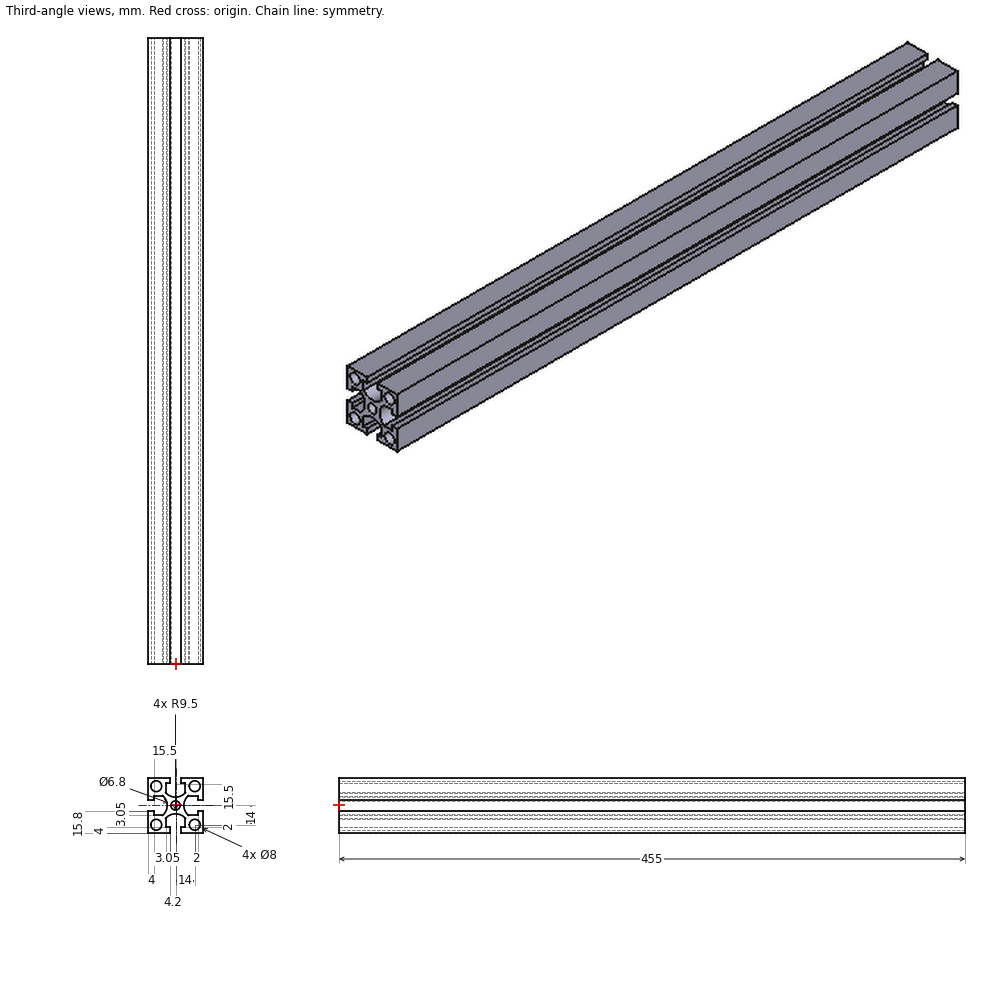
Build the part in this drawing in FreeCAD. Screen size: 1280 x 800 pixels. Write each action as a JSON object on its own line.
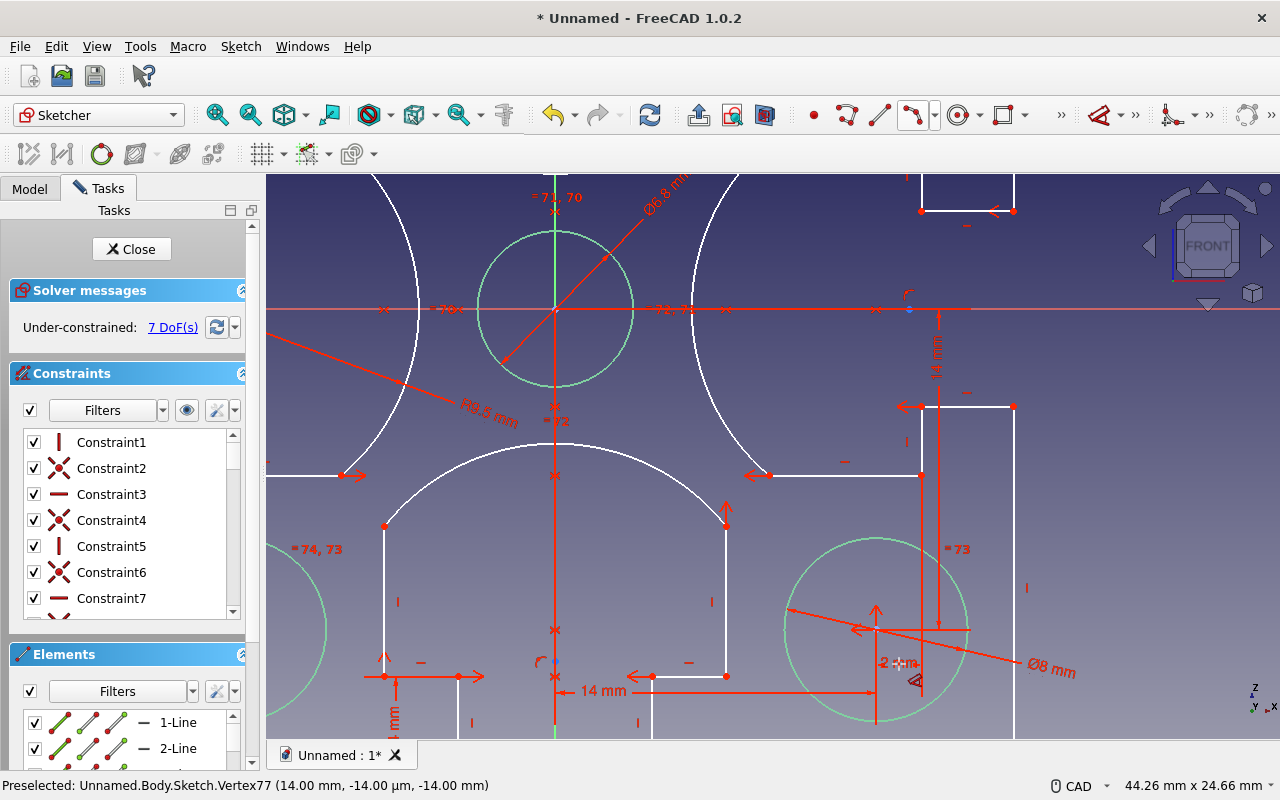
{"action": "left_click", "coordinate": [726, 677]}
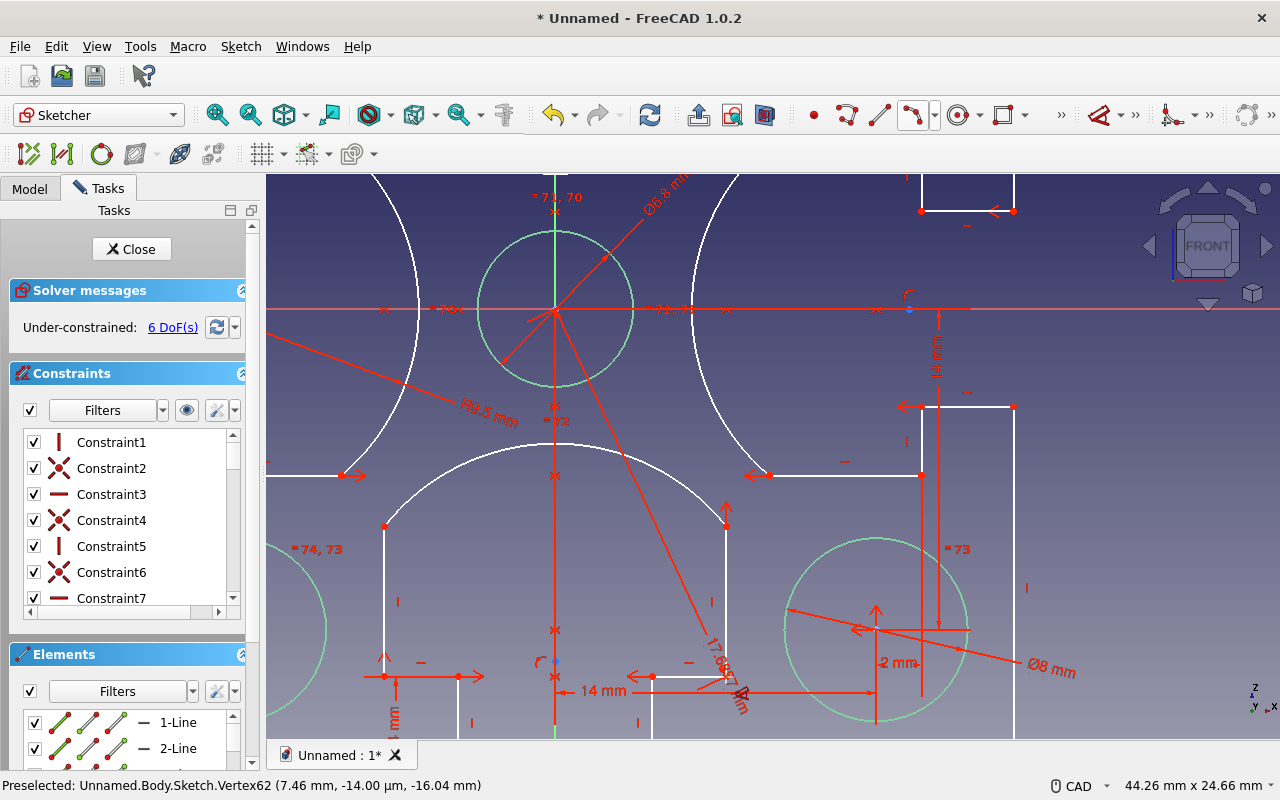
{"action": "left_click", "coordinate": [876, 630]}
{"action": "left_click", "coordinate": [910, 642]}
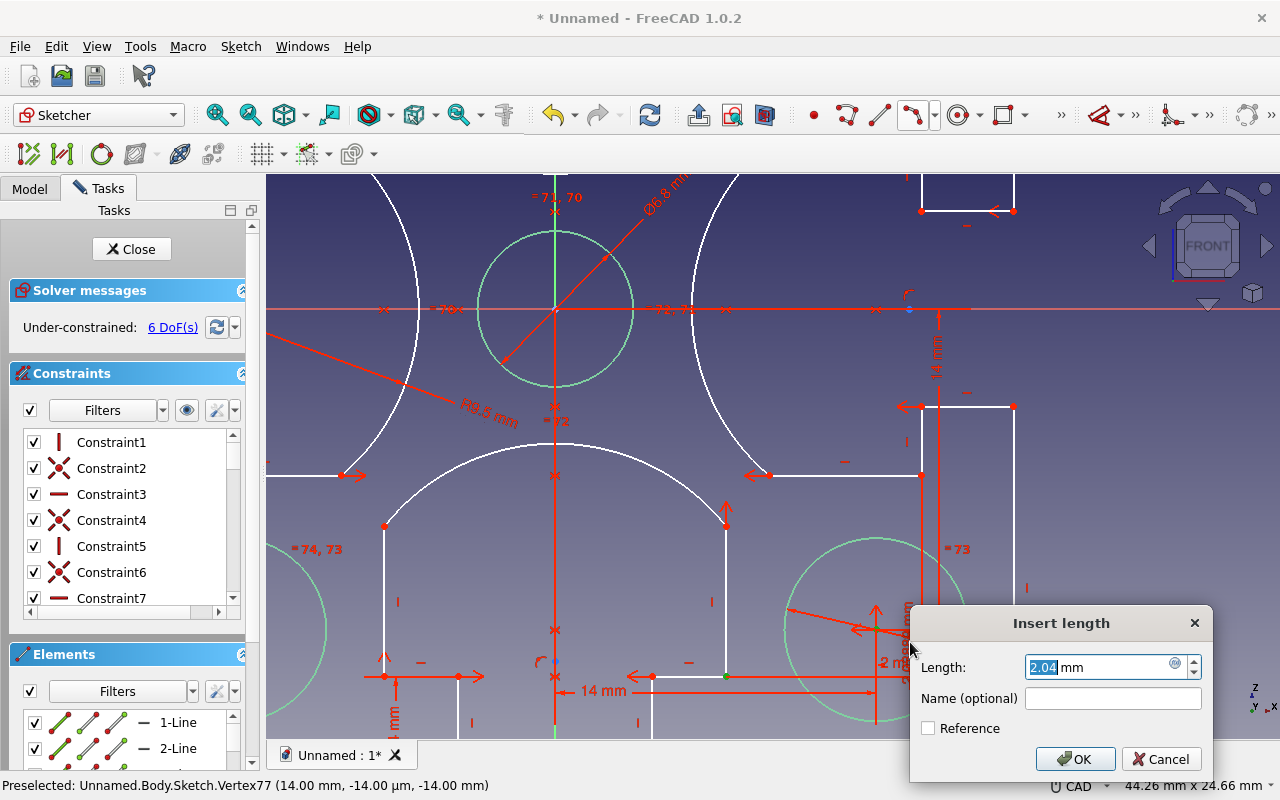
{"action": "type", "text": "2"}
{"action": "key", "text": "Return"}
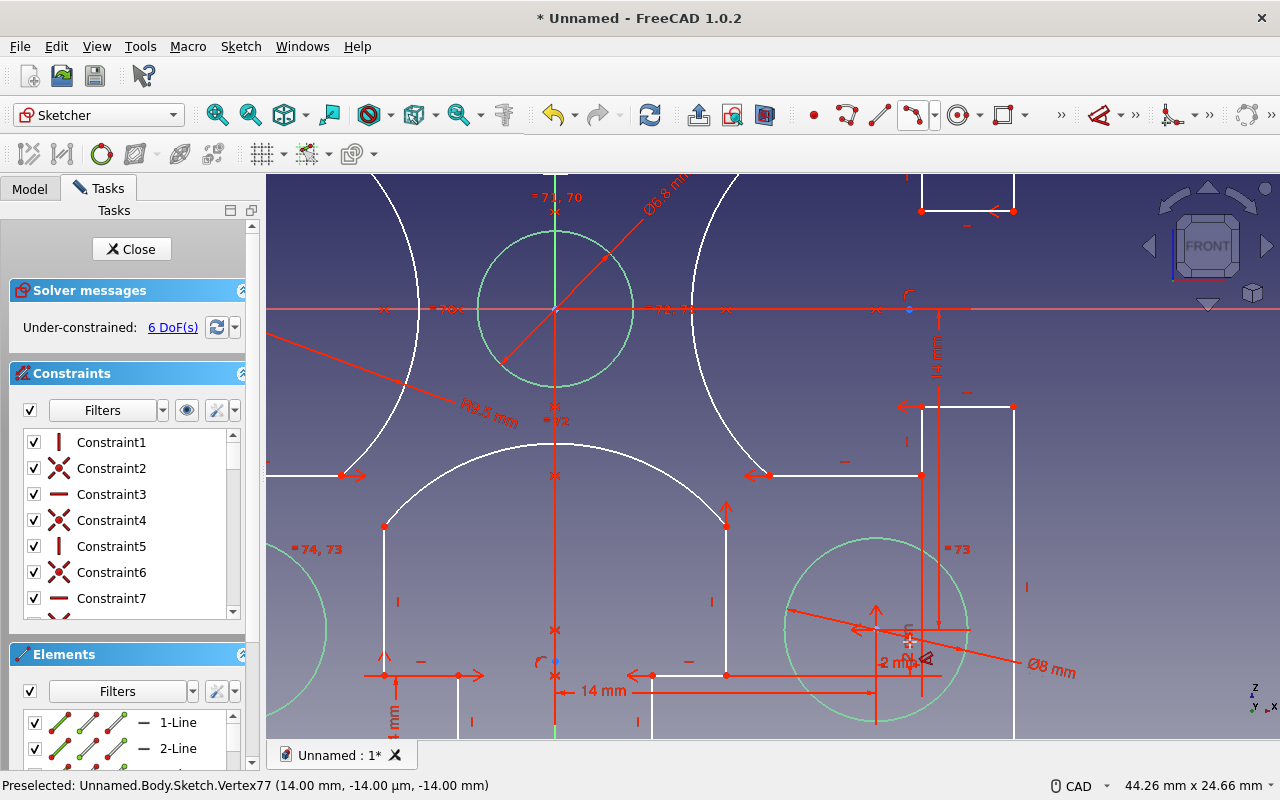
{"action": "left_click", "coordinate": [407, 676]}
{"action": "left_click", "coordinate": [421, 642]}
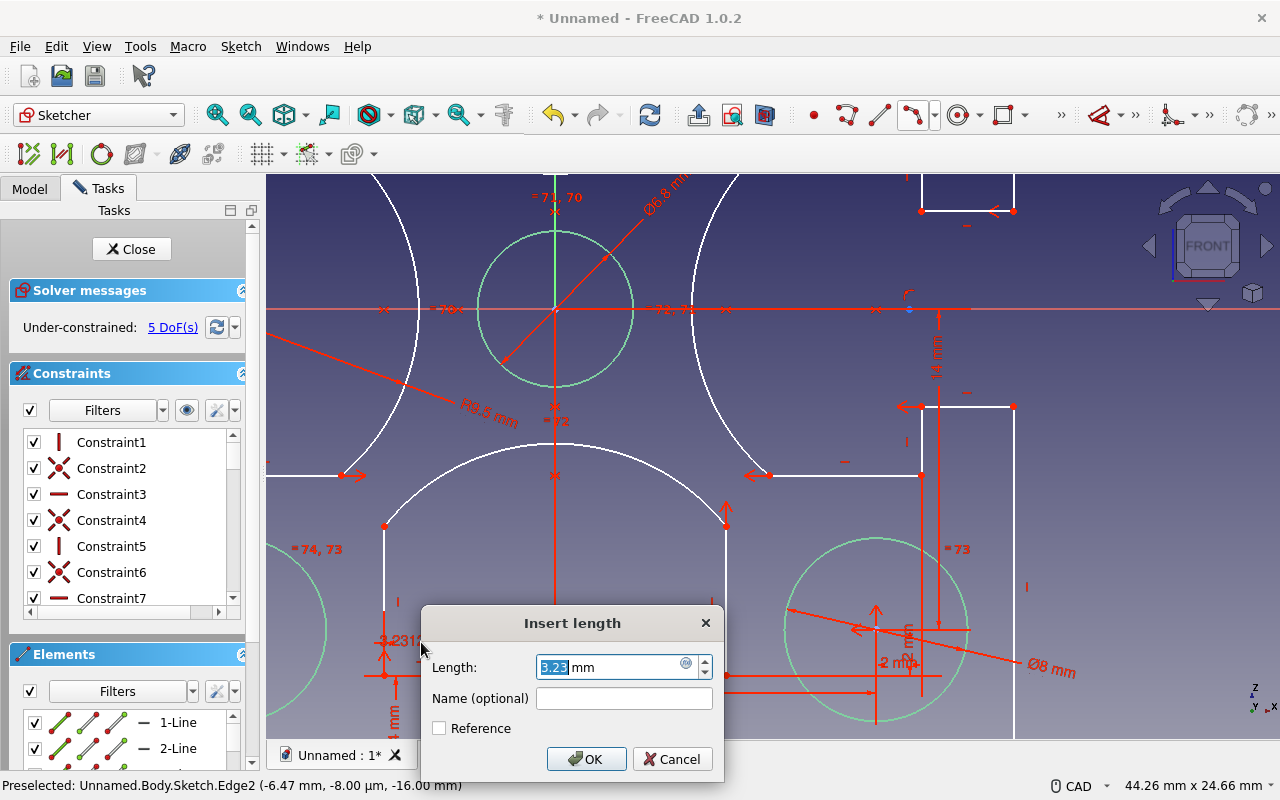
{"action": "type", "text": "3.05"}
{"action": "key", "text": "Return"}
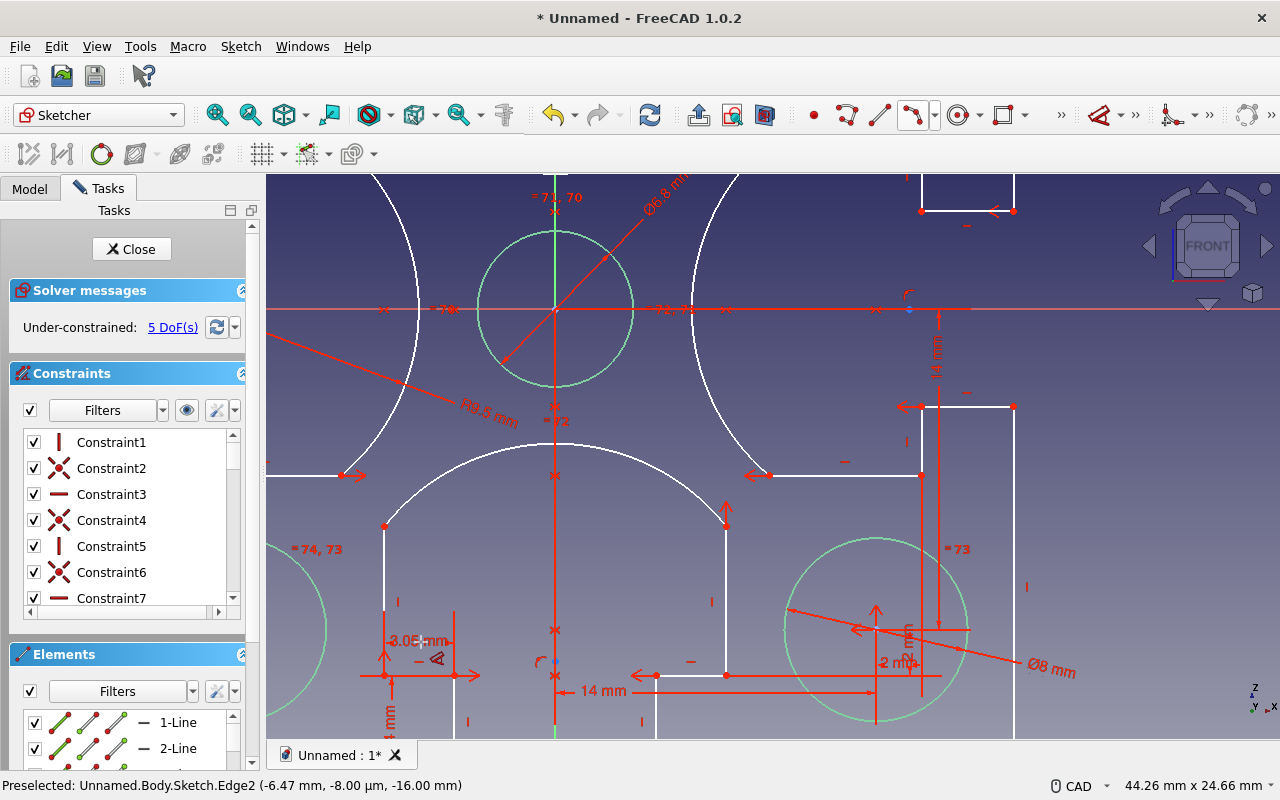
{"action": "scroll", "coordinate": [791, 542], "scroll_direction": "down", "scroll_amount": 5}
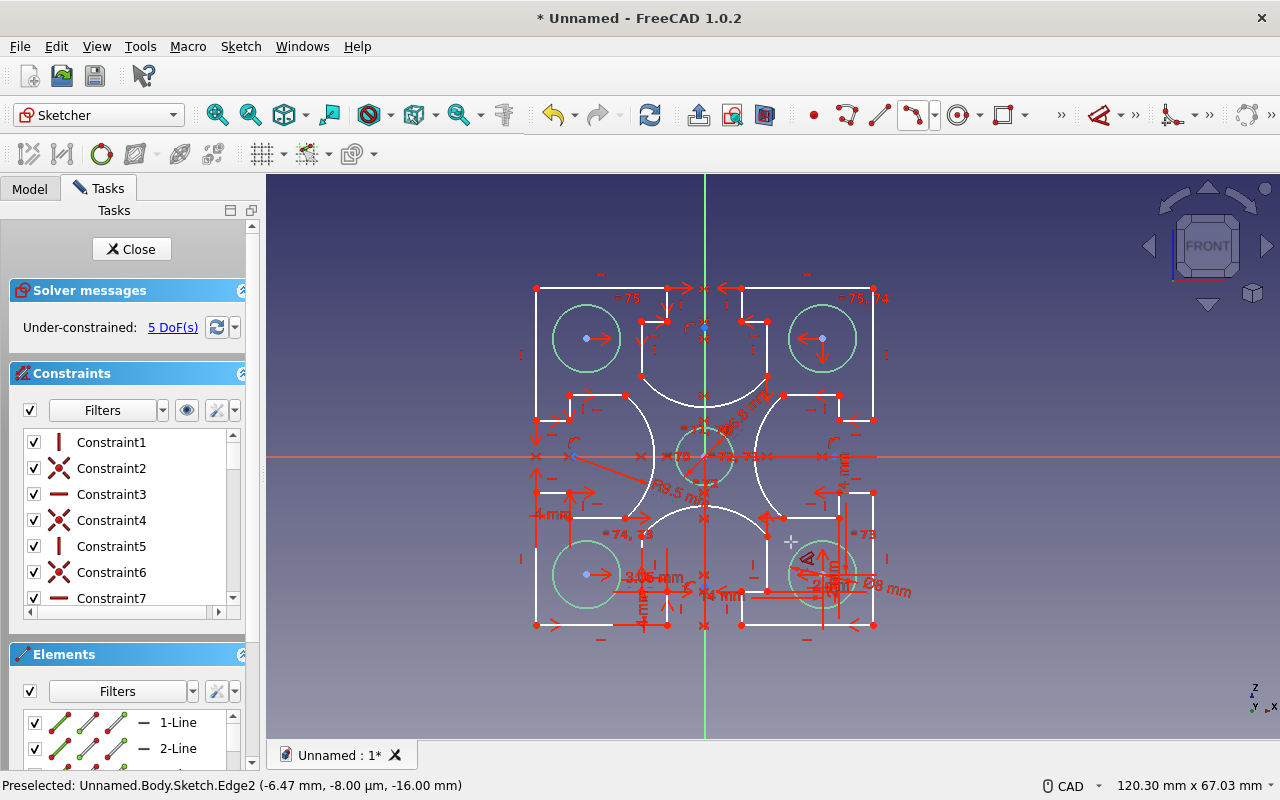
{"action": "left_click", "coordinate": [536, 585]}
{"action": "left_click", "coordinate": [502, 559]}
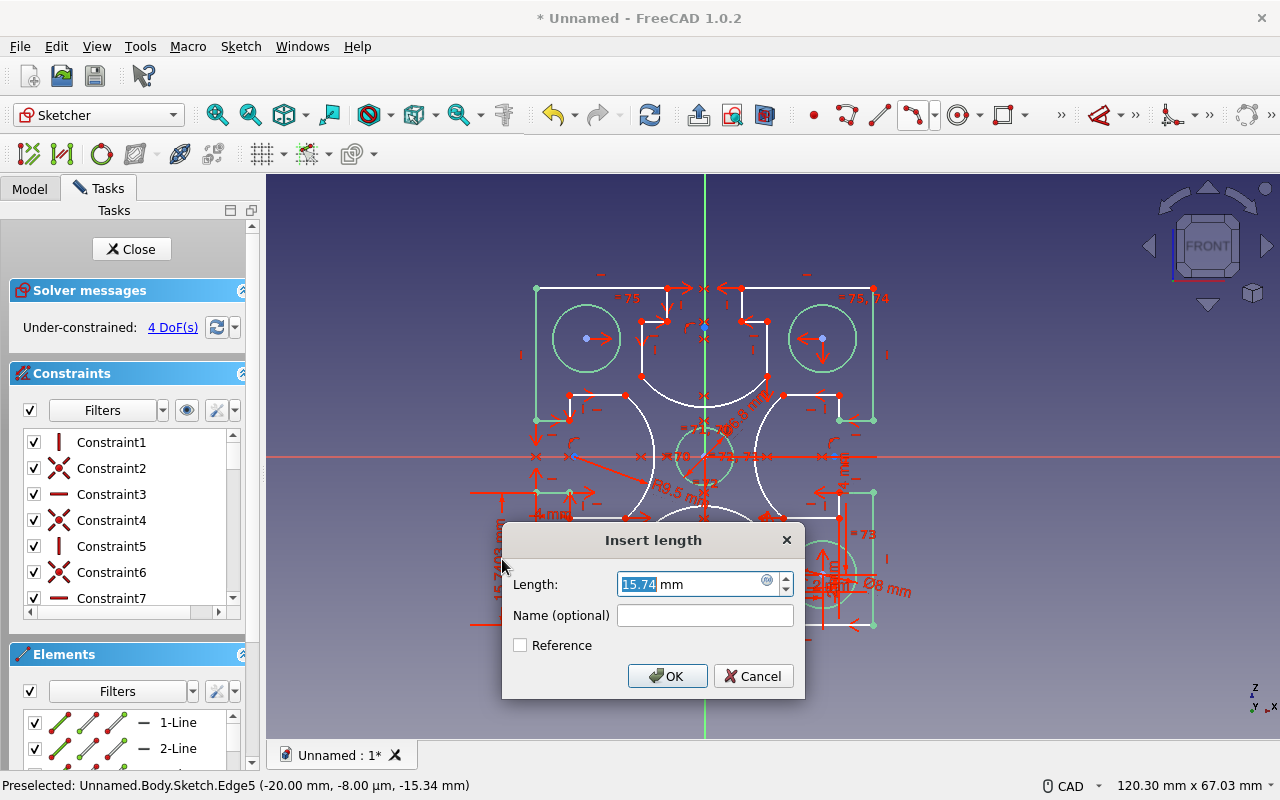
{"action": "type", "text": "15.8"}
{"action": "key", "text": "Return"}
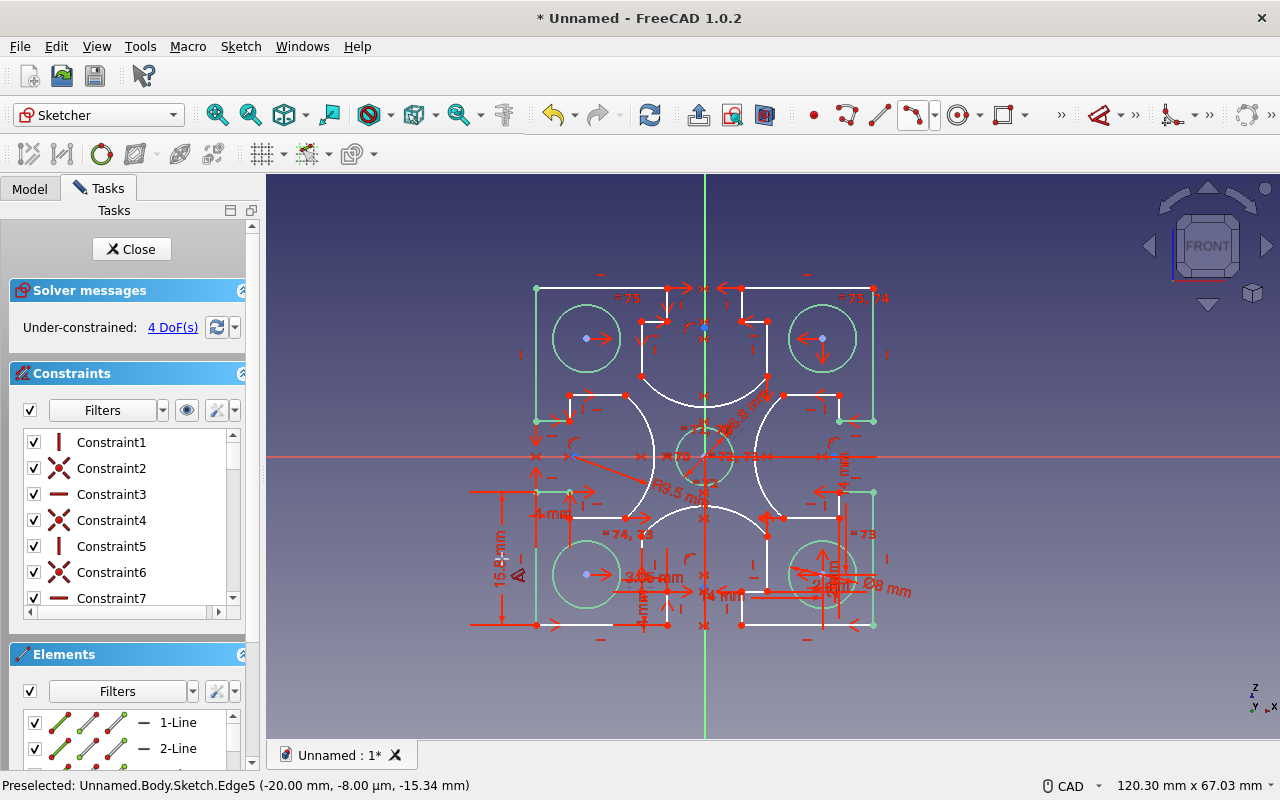
{"action": "scroll", "coordinate": [570, 502], "scroll_direction": "up", "scroll_amount": 3}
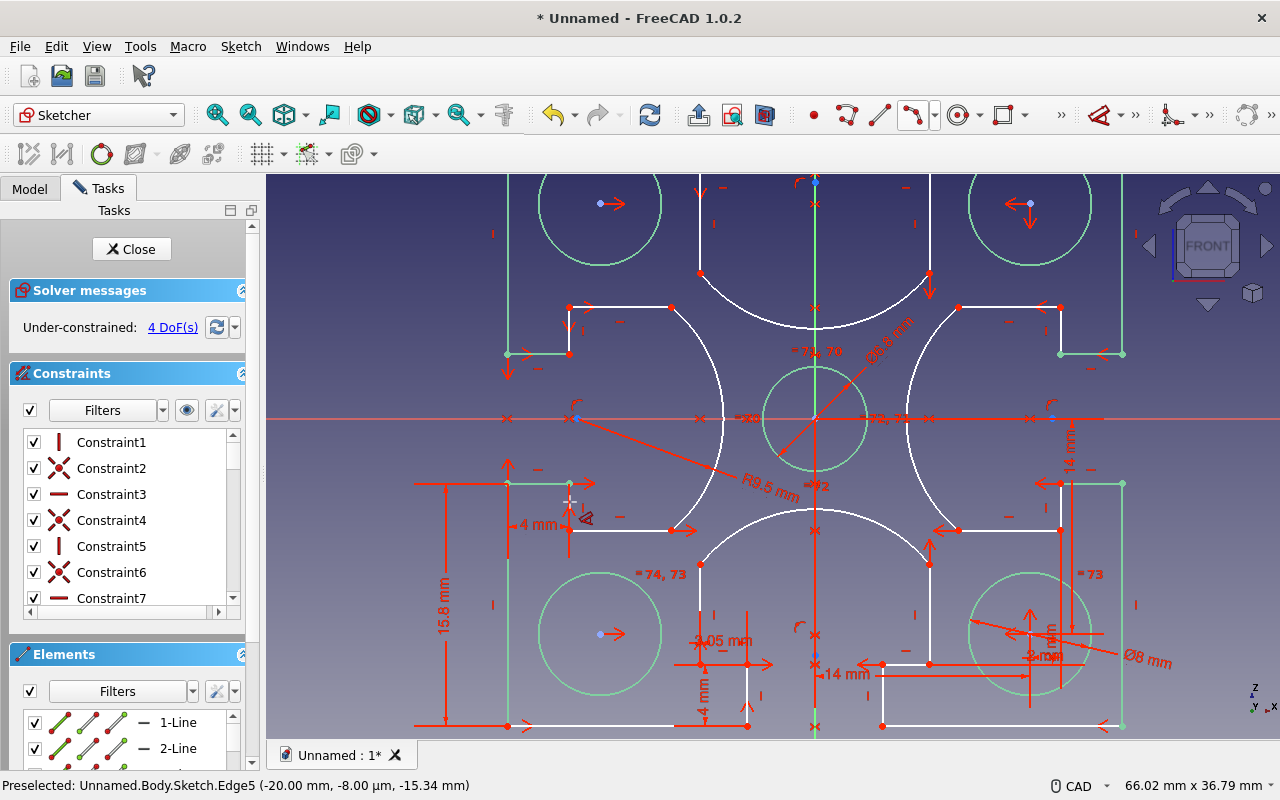
{"action": "left_click", "coordinate": [569, 502]}
{"action": "left_click", "coordinate": [603, 496]}